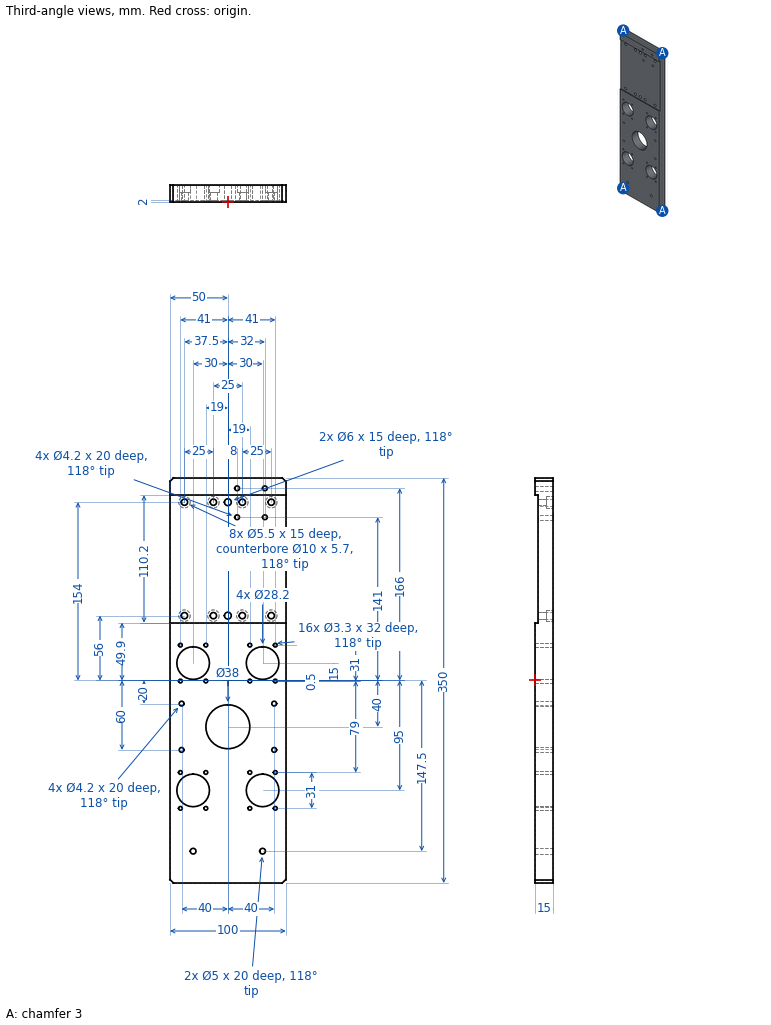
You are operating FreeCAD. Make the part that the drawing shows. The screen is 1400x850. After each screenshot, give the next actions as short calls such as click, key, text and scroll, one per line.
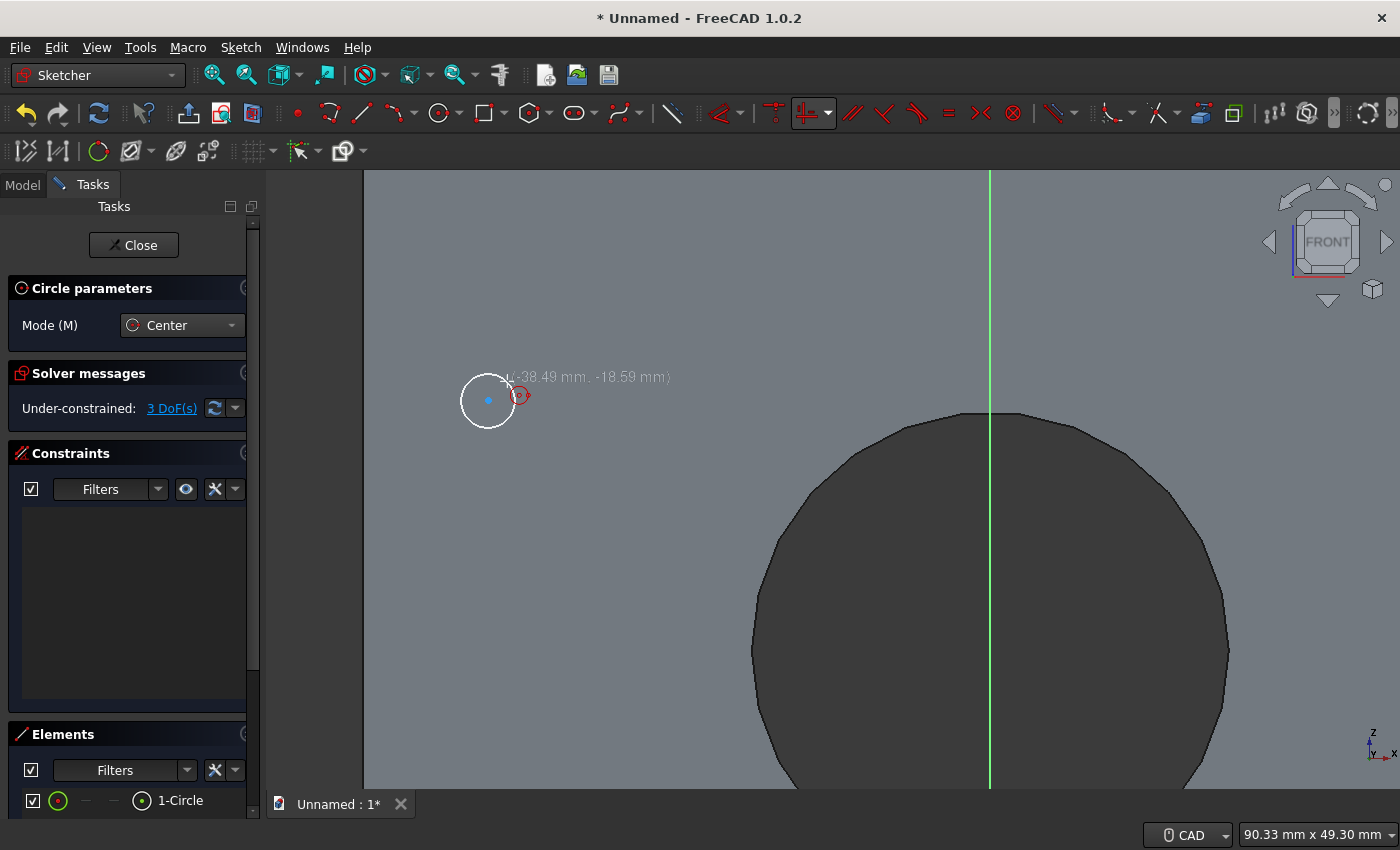
scroll(490, 408, down, 3)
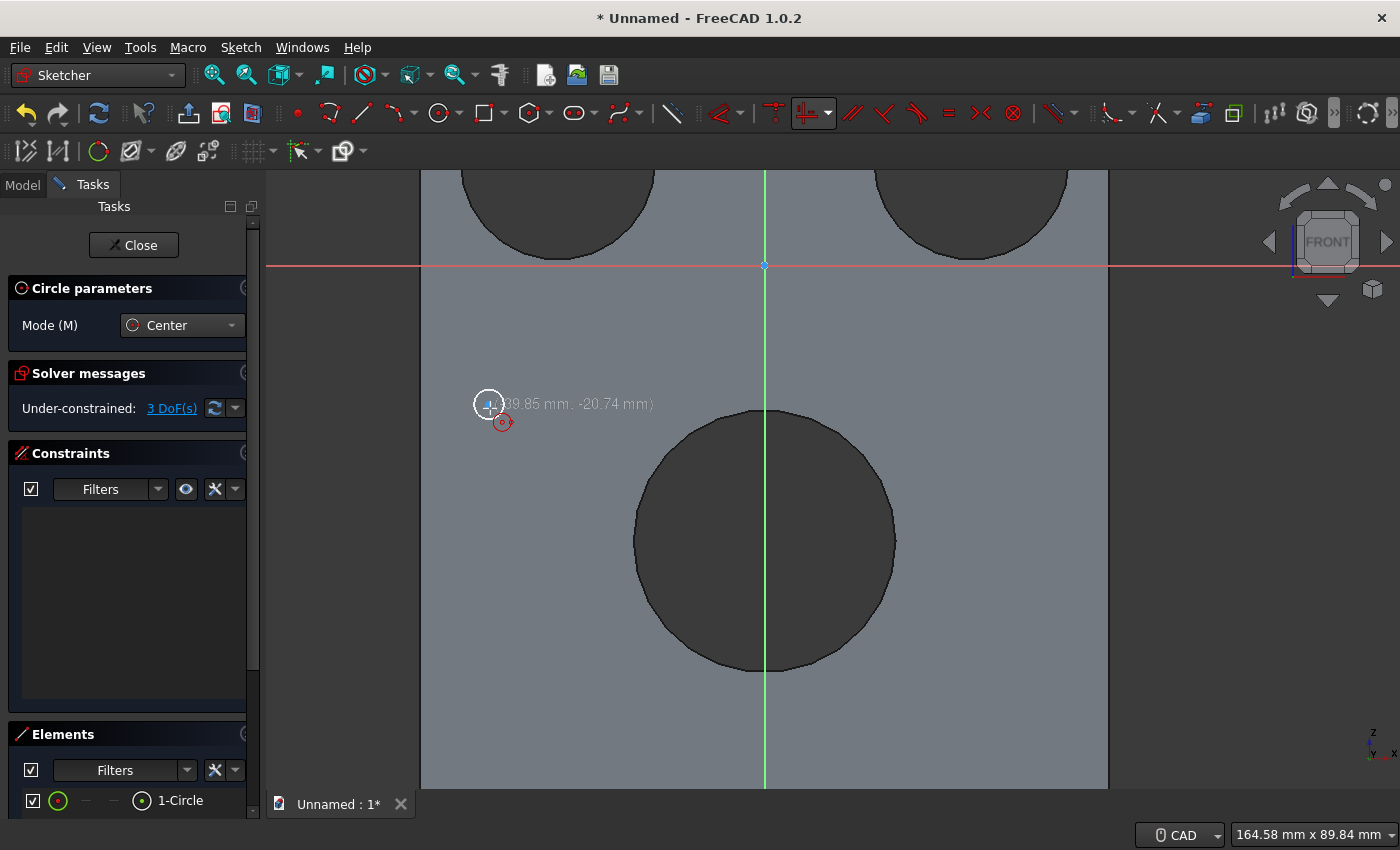
scroll(1040, 404, up, 3)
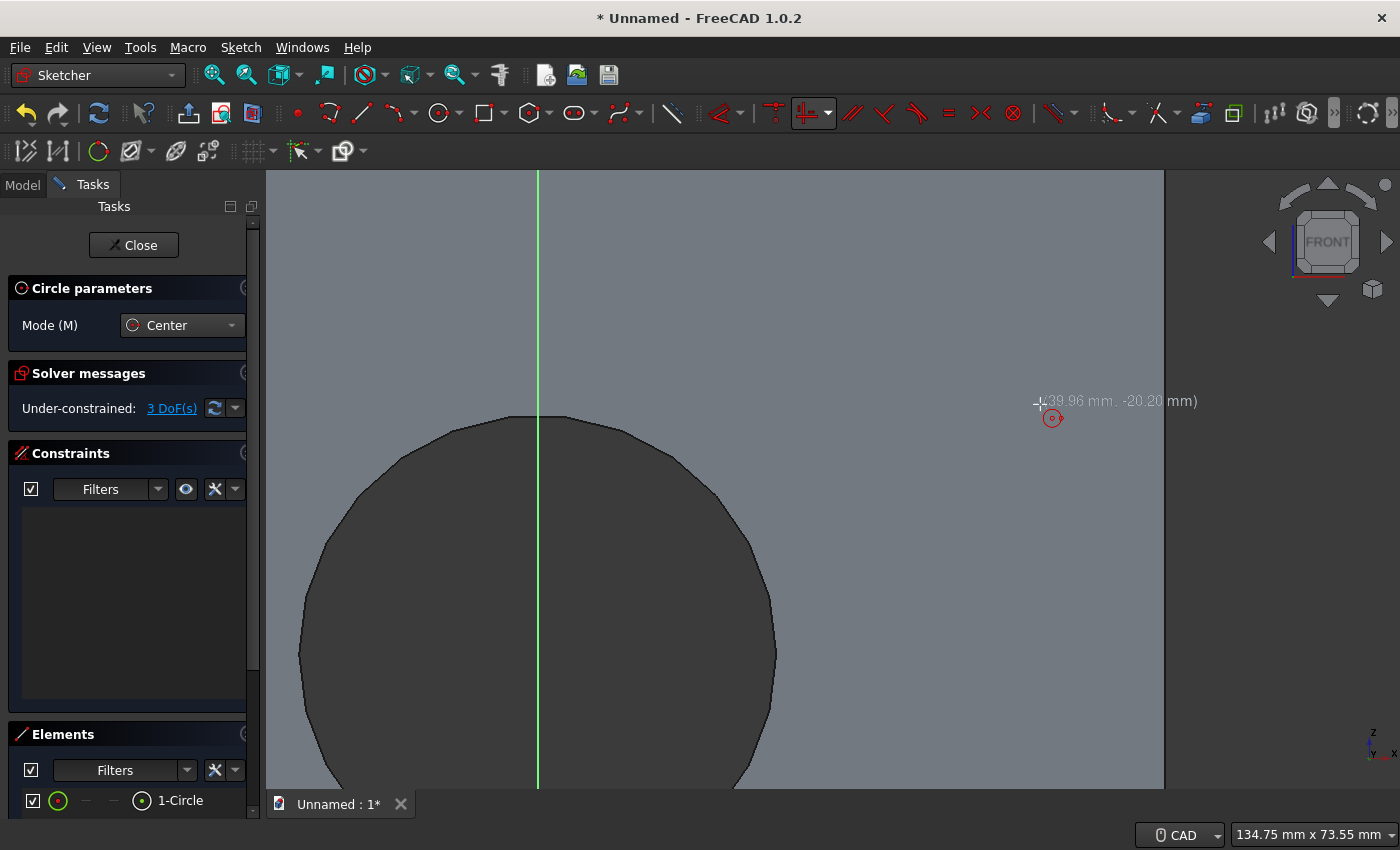
click(1040, 403)
click(1059, 384)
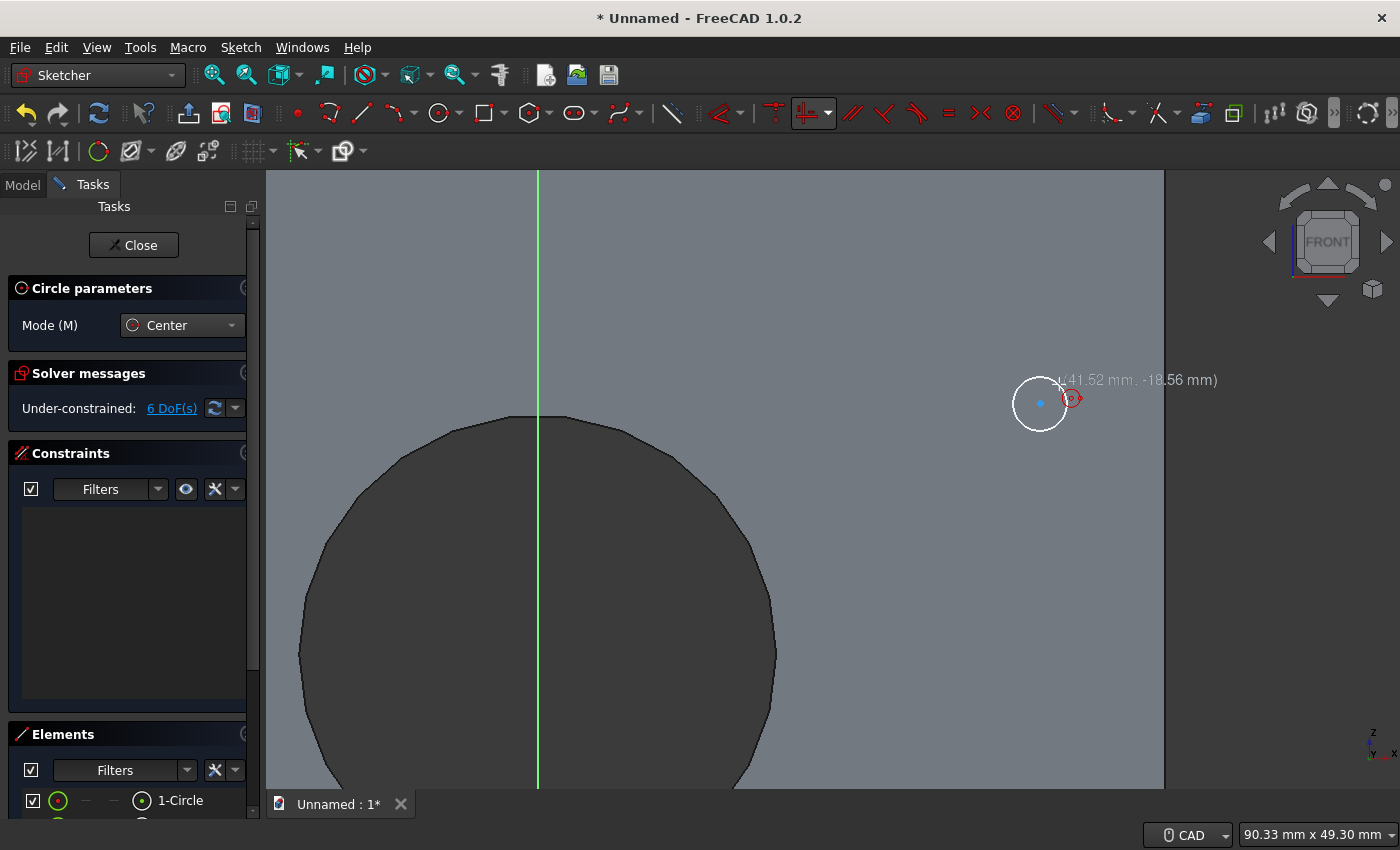
scroll(1040, 404, down, 3)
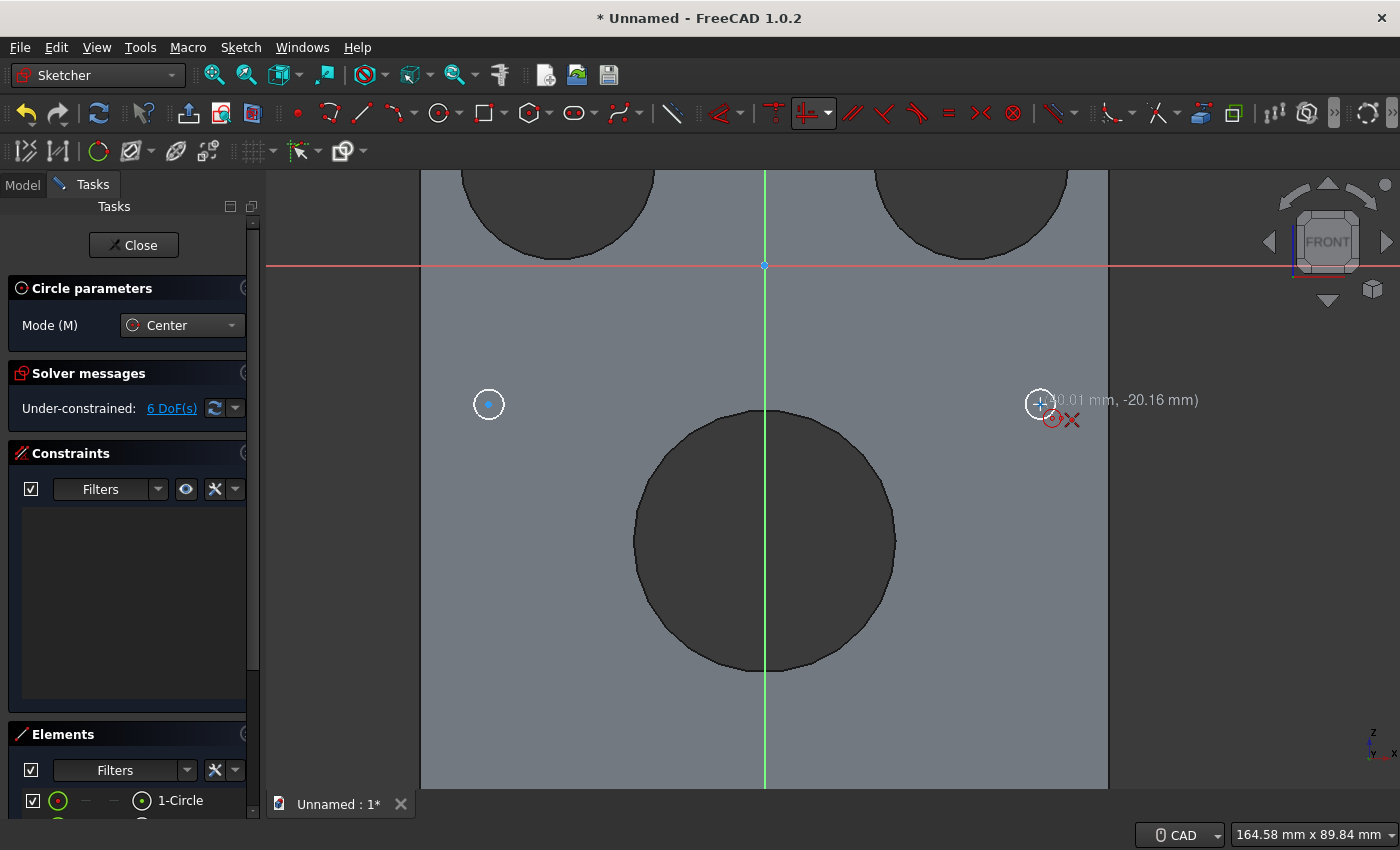
scroll(489, 679, up, 3)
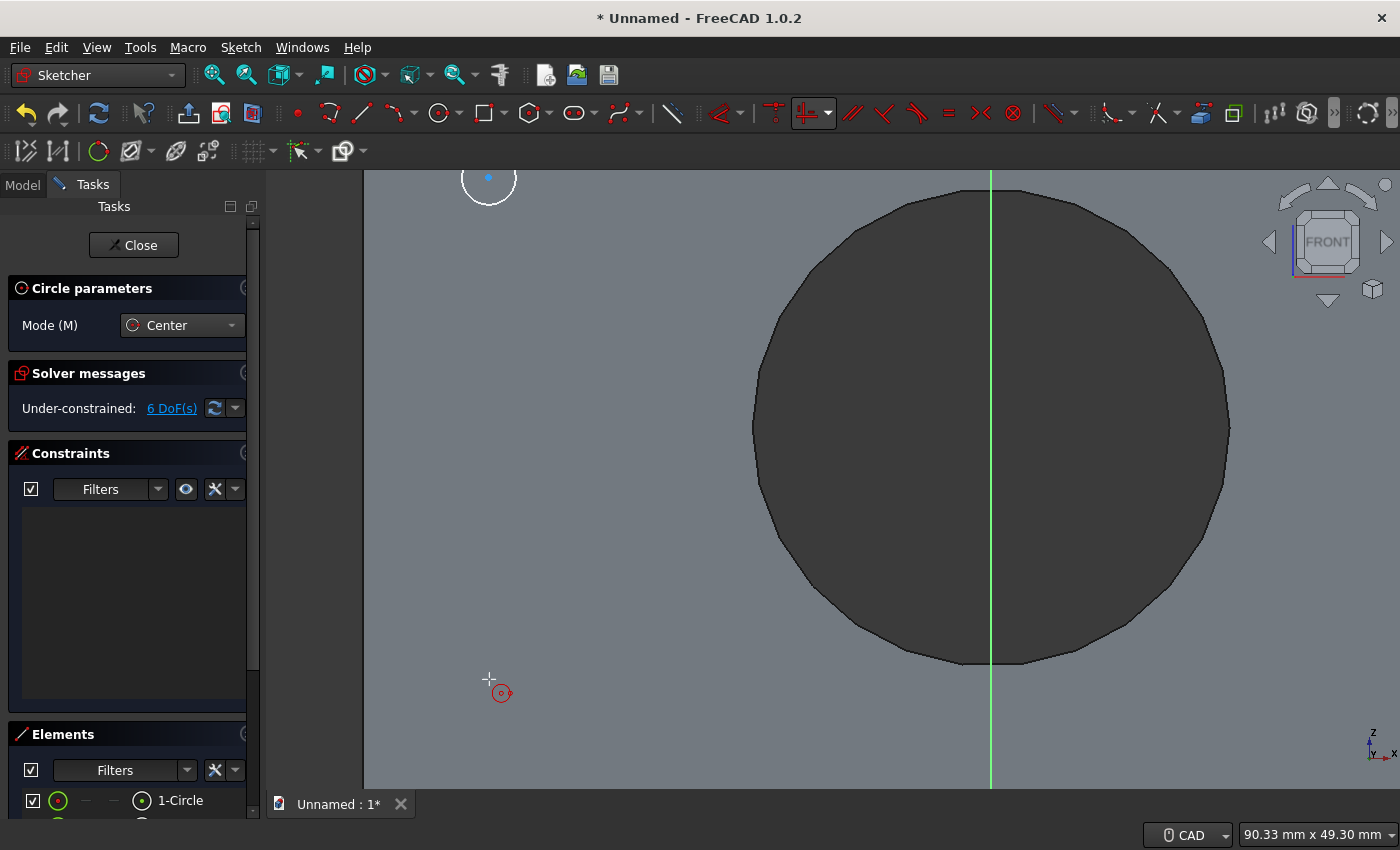
click(489, 679)
click(508, 660)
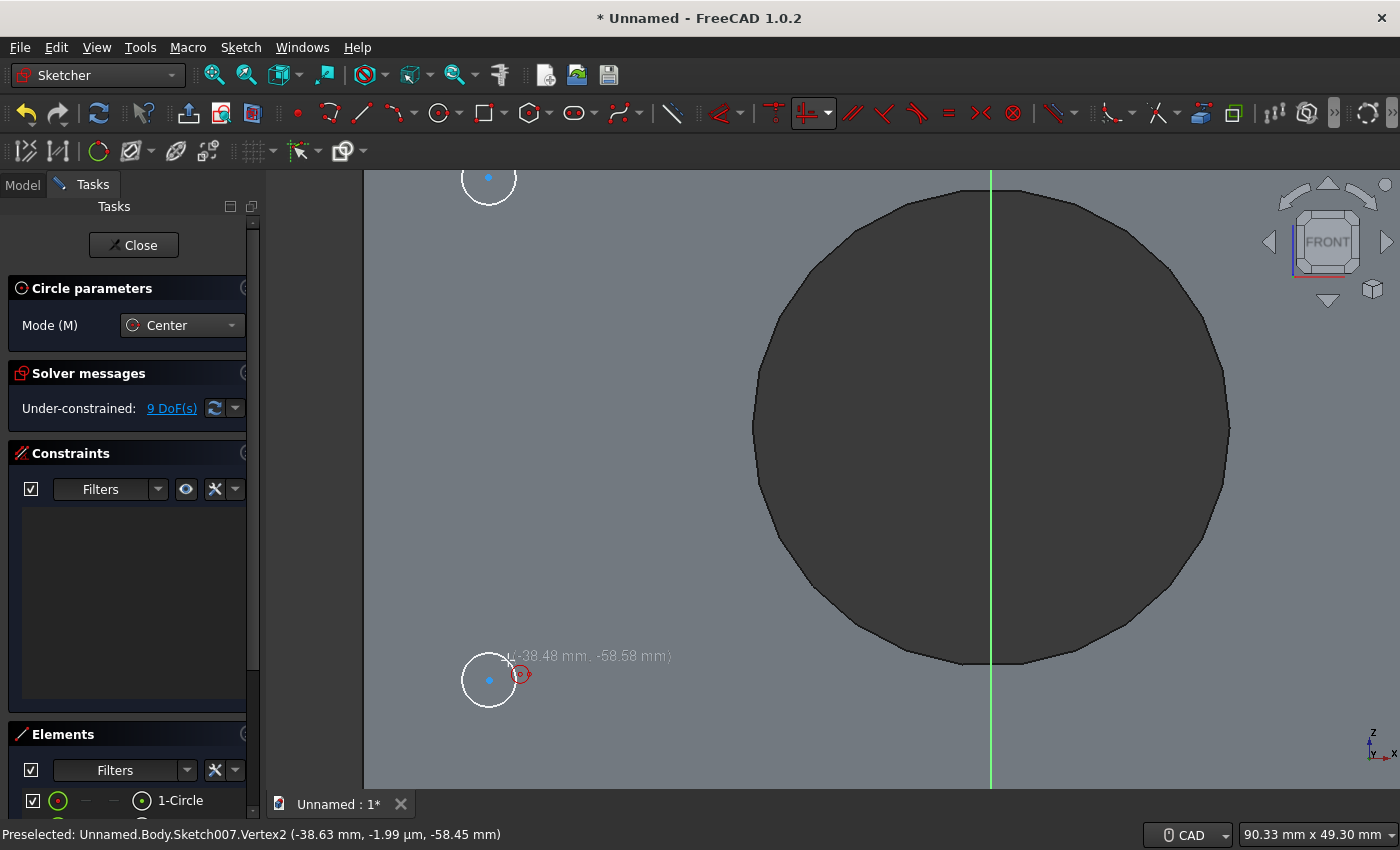
scroll(489, 679, down, 3)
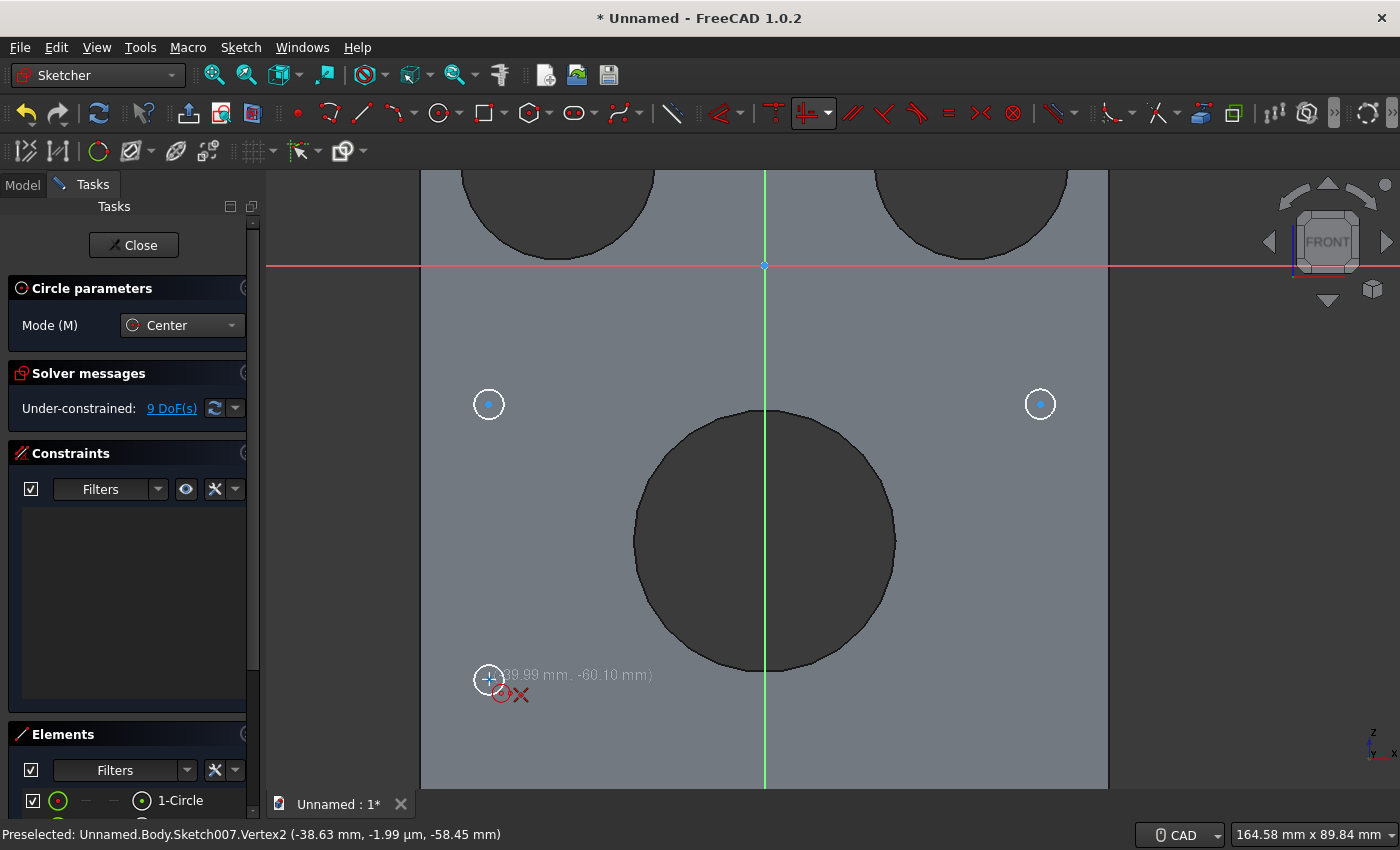
scroll(1040, 679, up, 3)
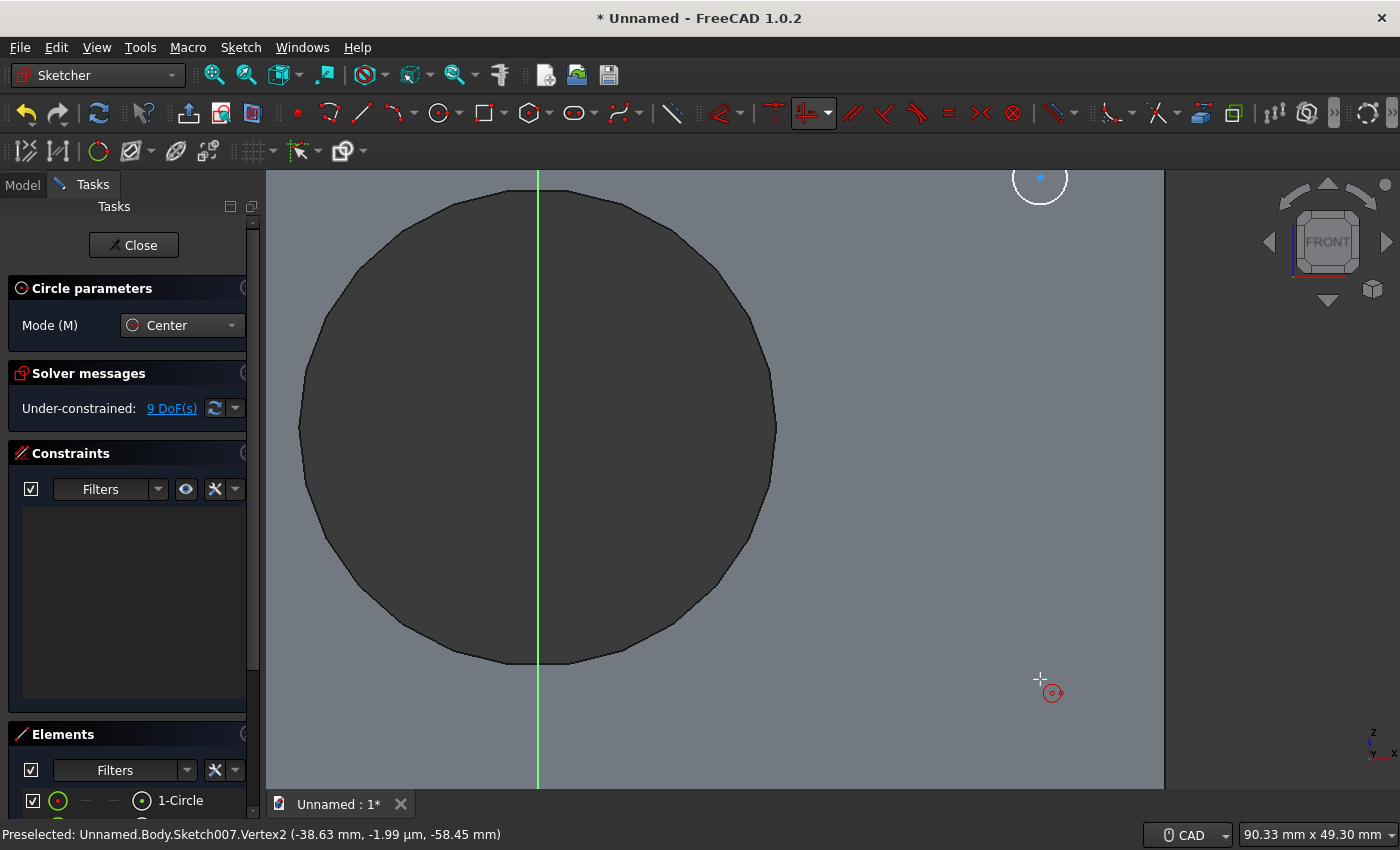
click(1040, 679)
click(1059, 660)
key(Escape)